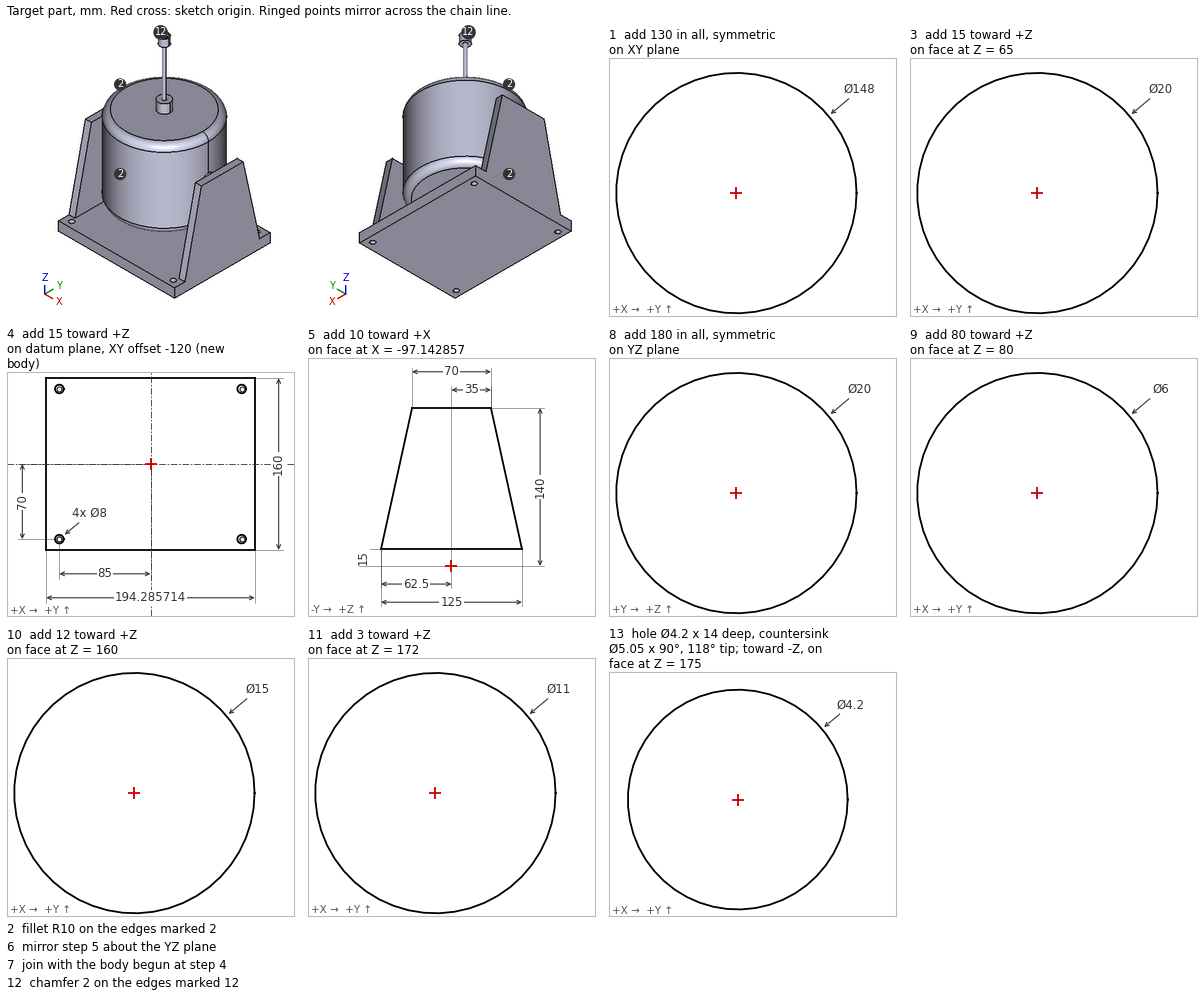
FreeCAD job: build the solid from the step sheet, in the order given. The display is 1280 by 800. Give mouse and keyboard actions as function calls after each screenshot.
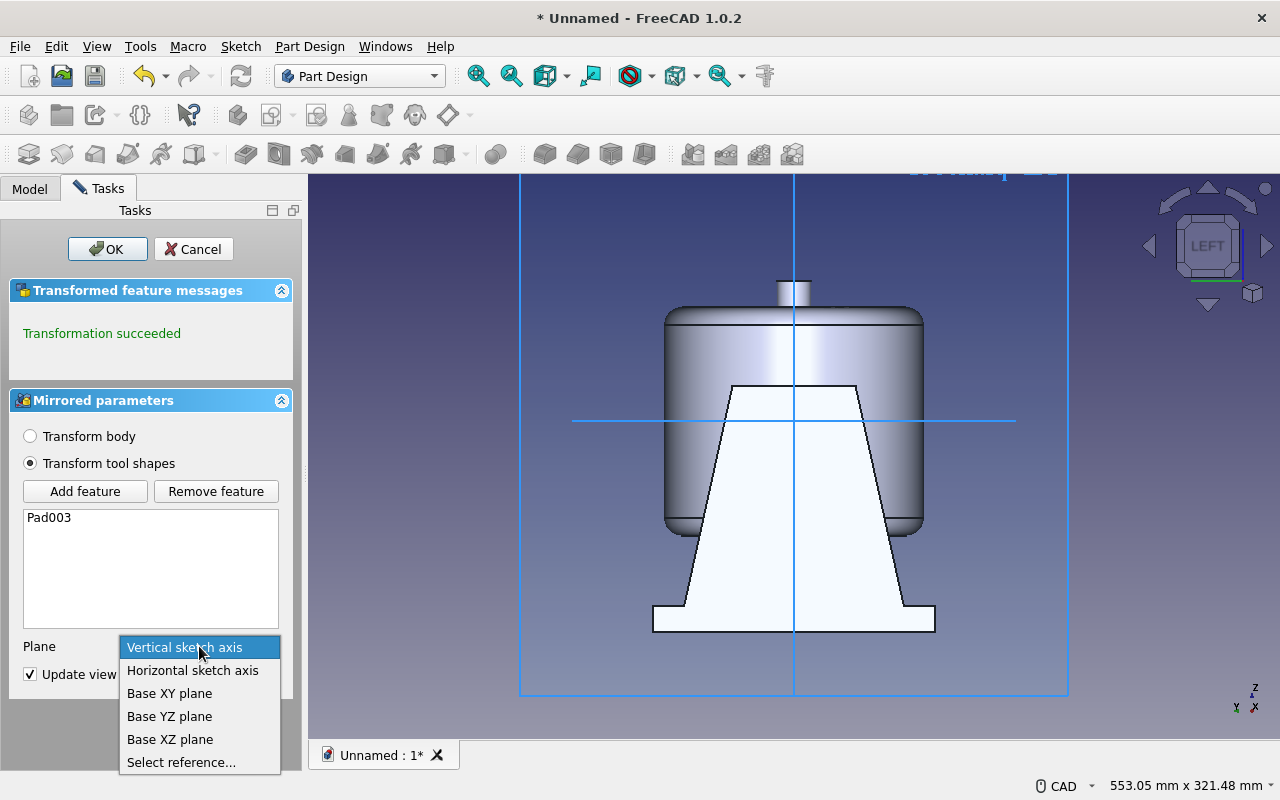
click(198, 716)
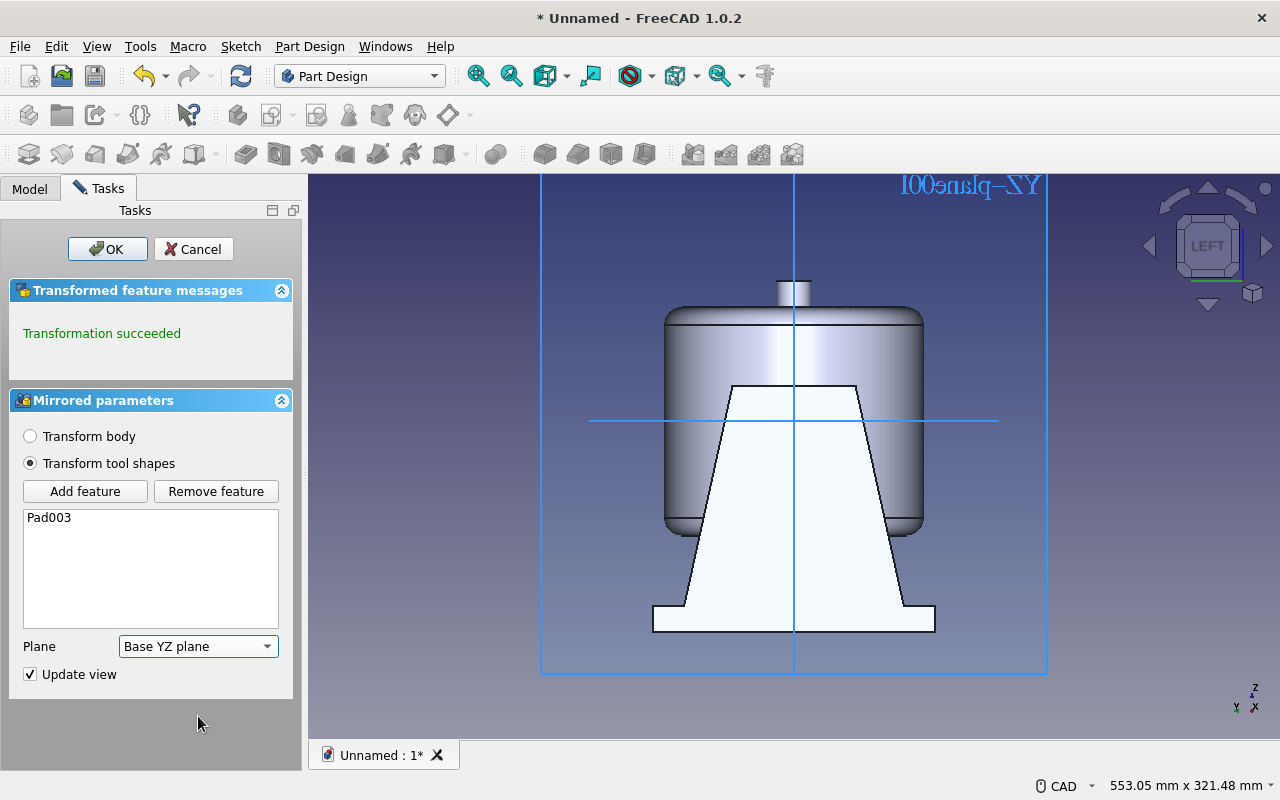
click(108, 249)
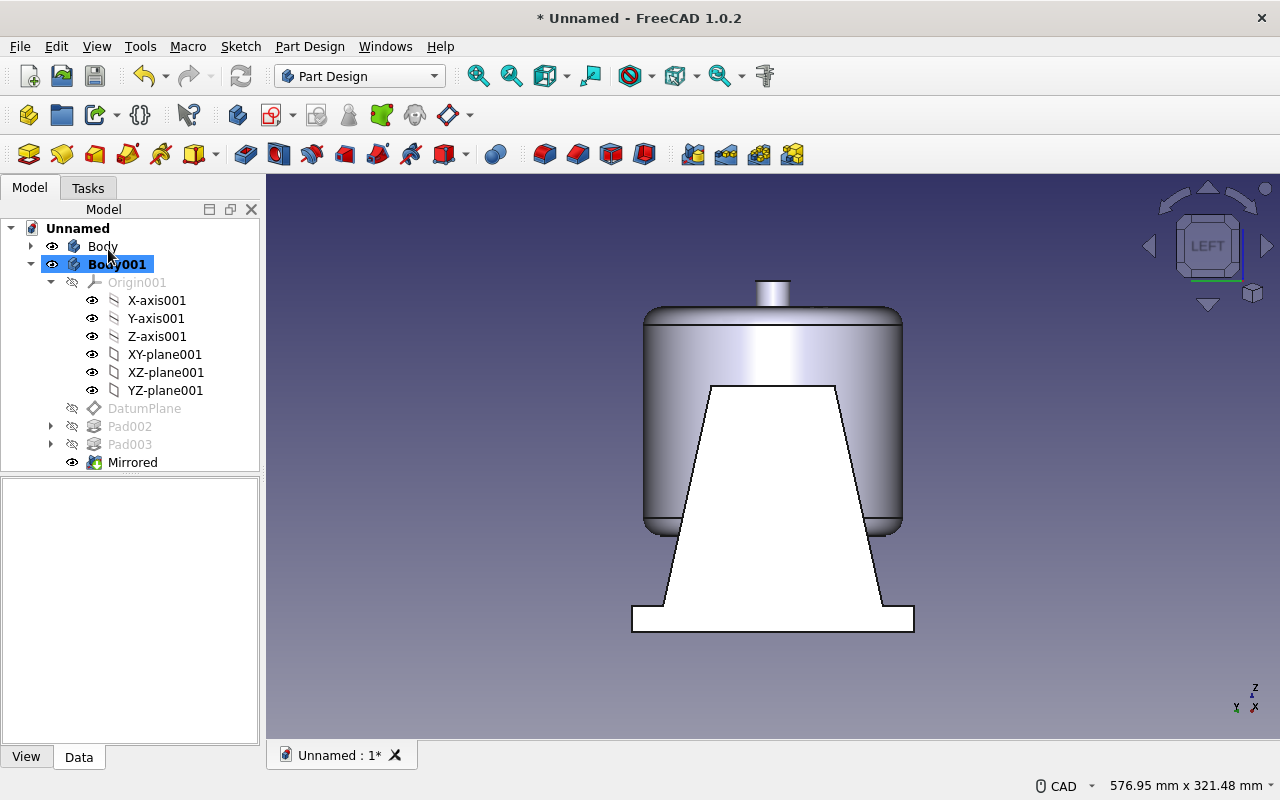
key(v)
key(f)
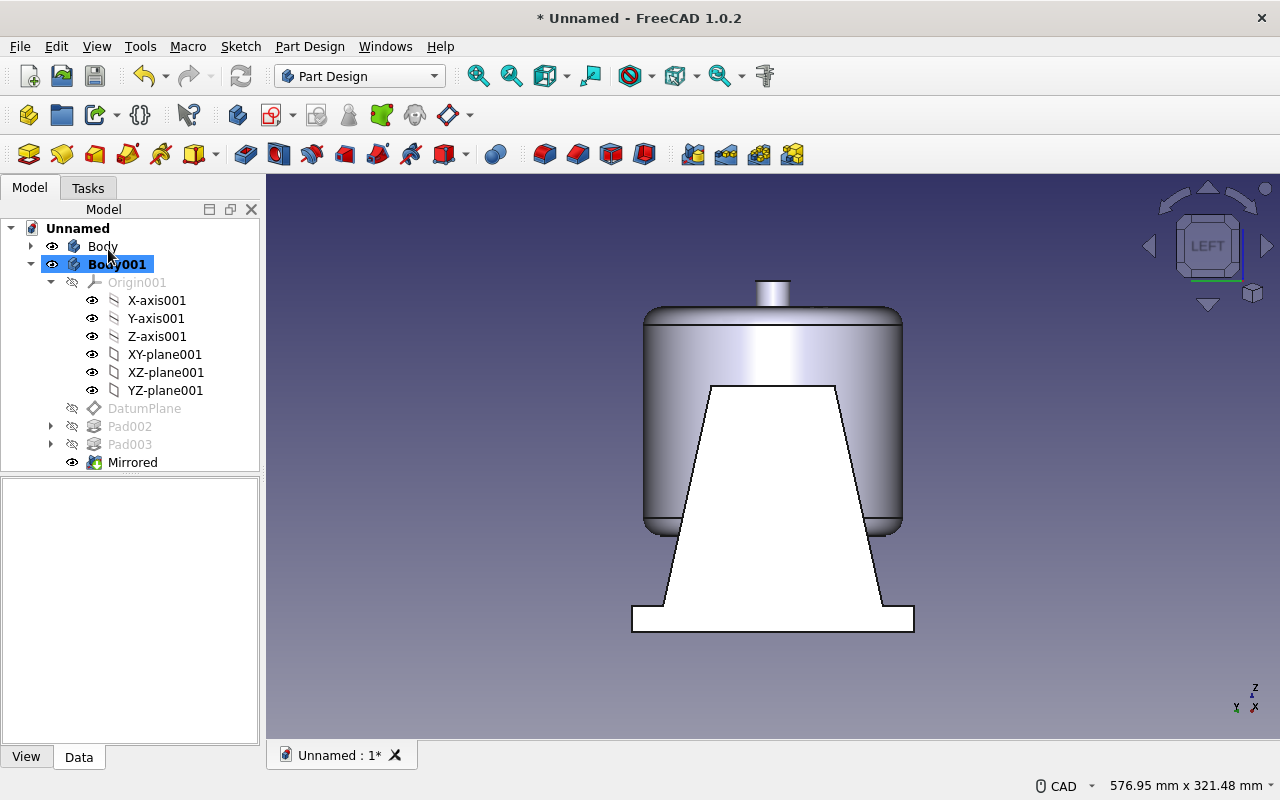
double_click(97, 246)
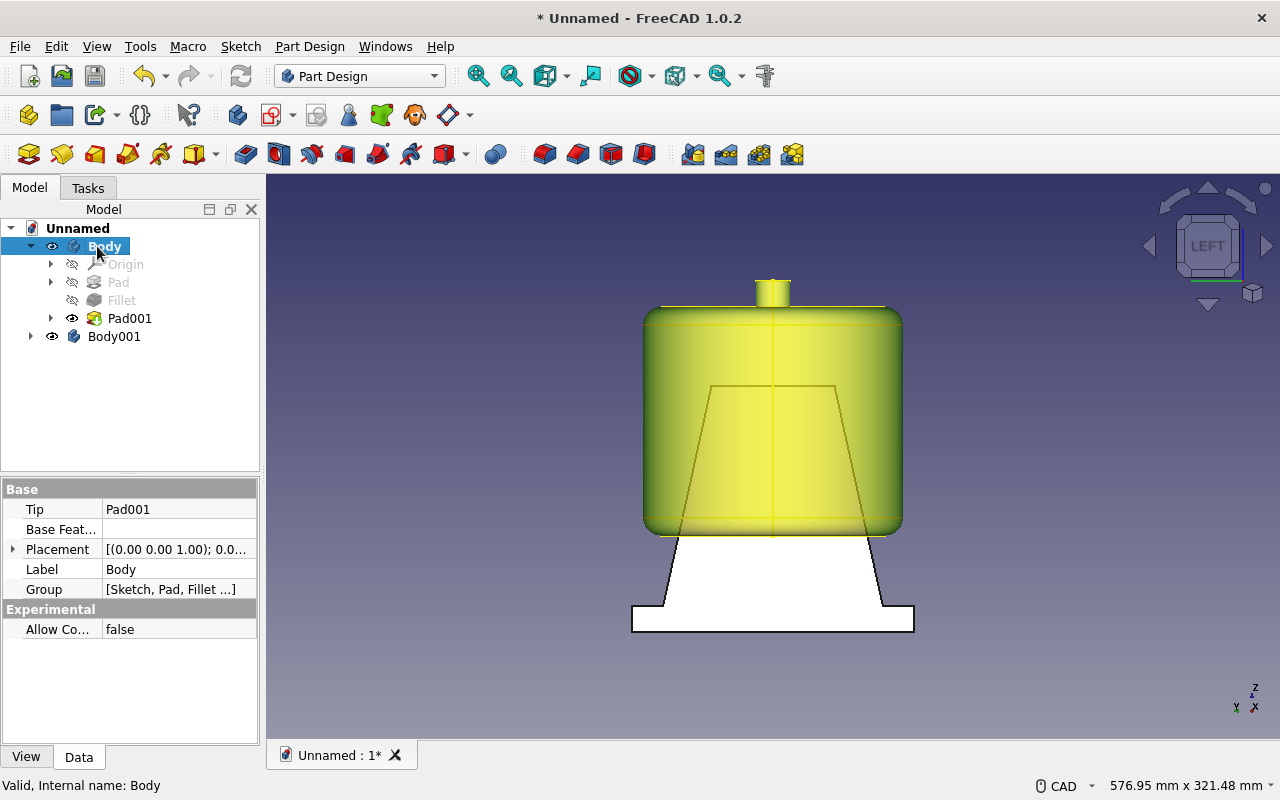
click(97, 246)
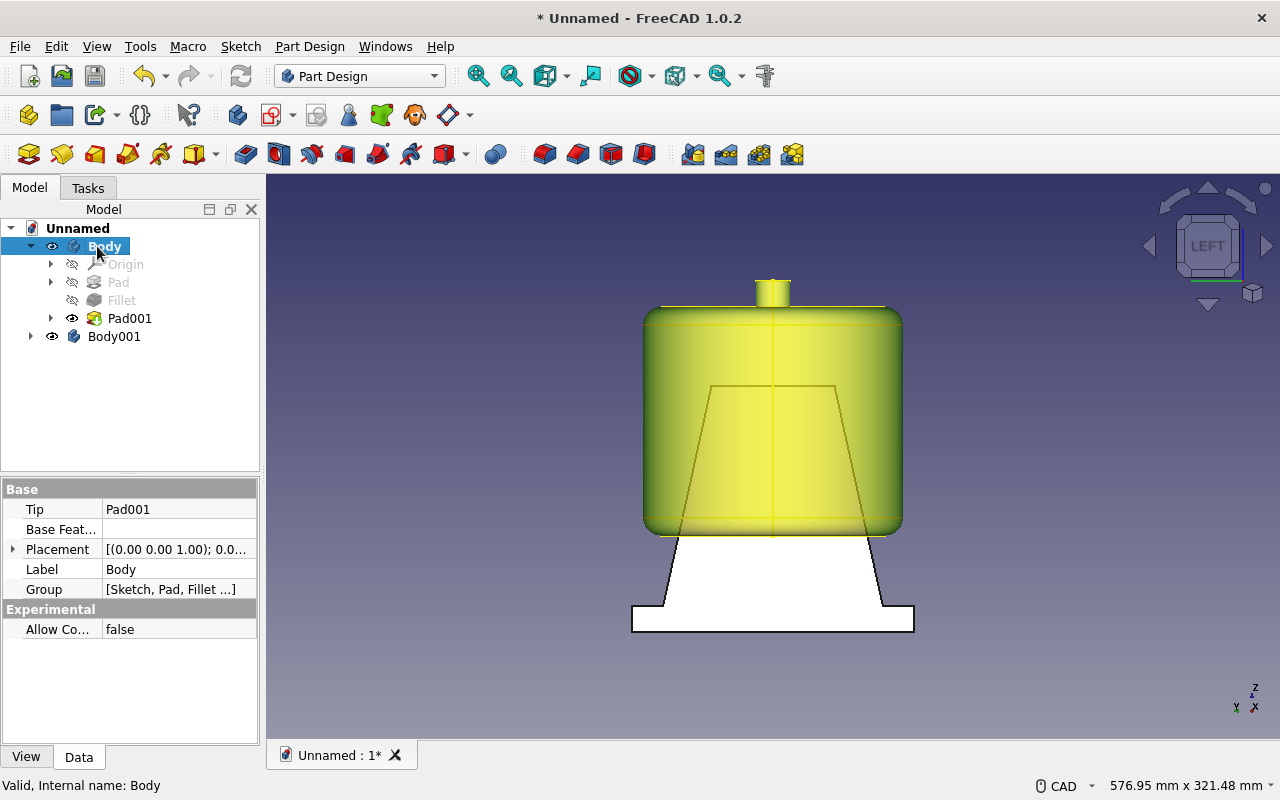
click(148, 629)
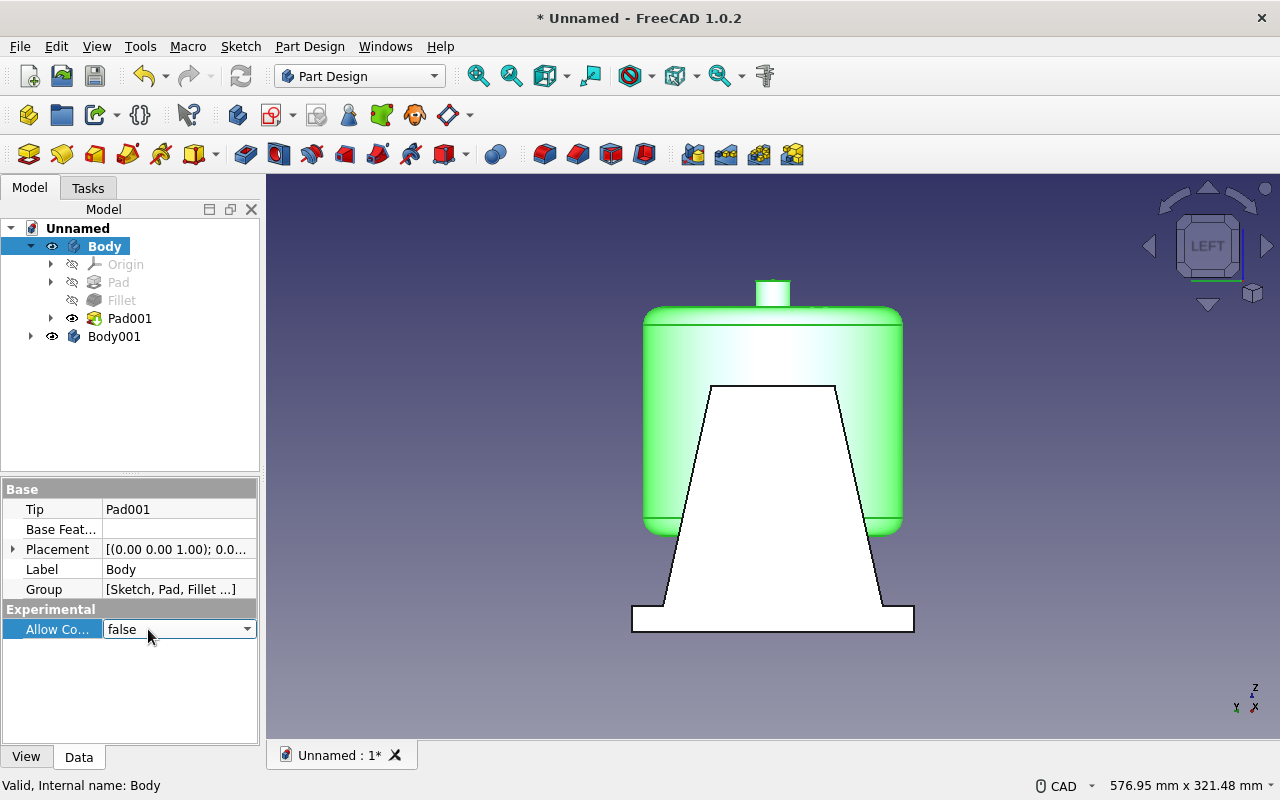
click(148, 629)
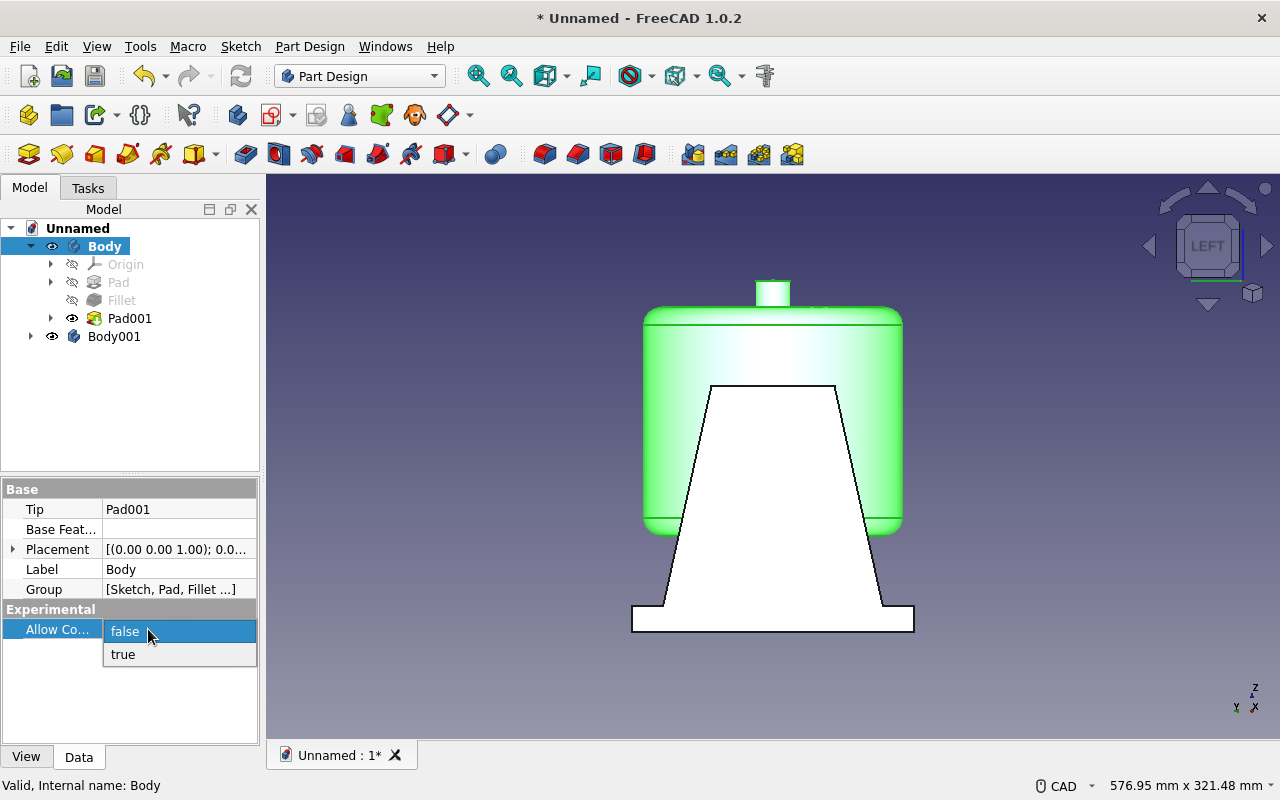
click(178, 654)
key(Return)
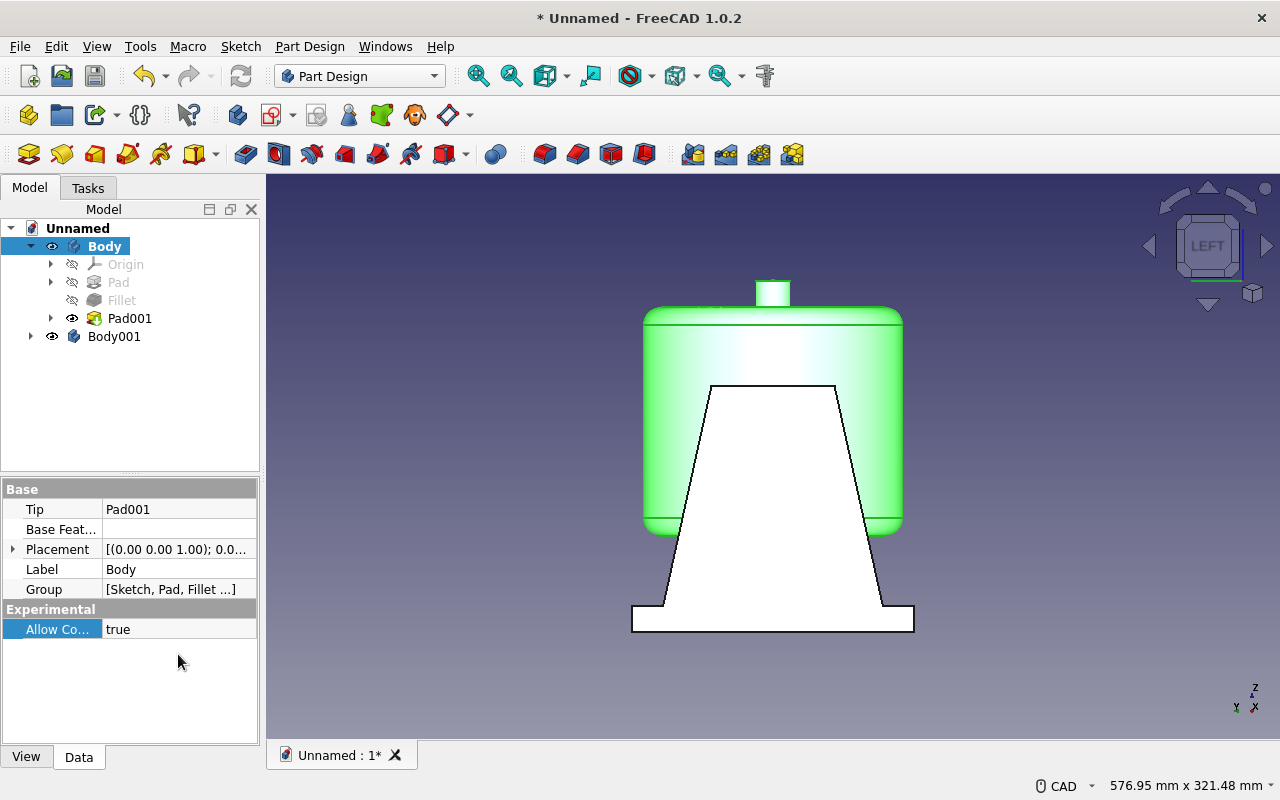
click(97, 336)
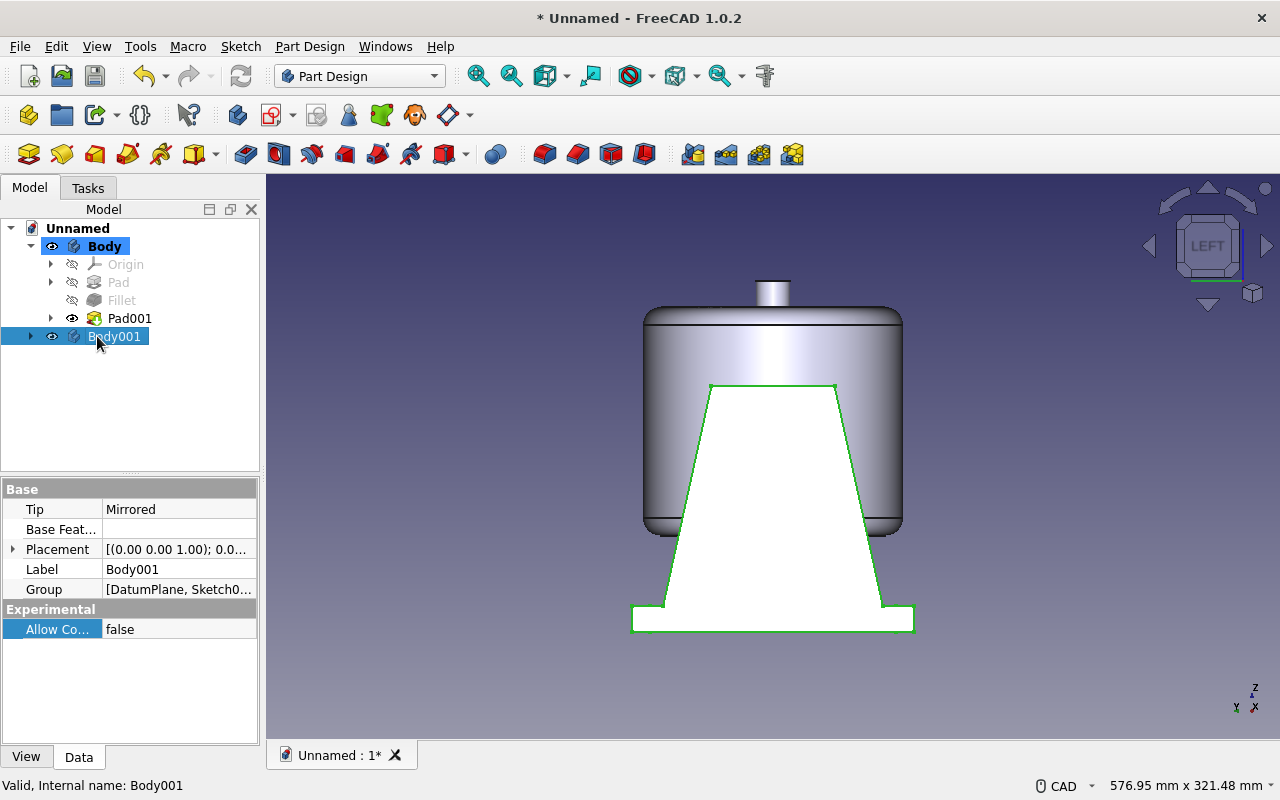
click(496, 154)